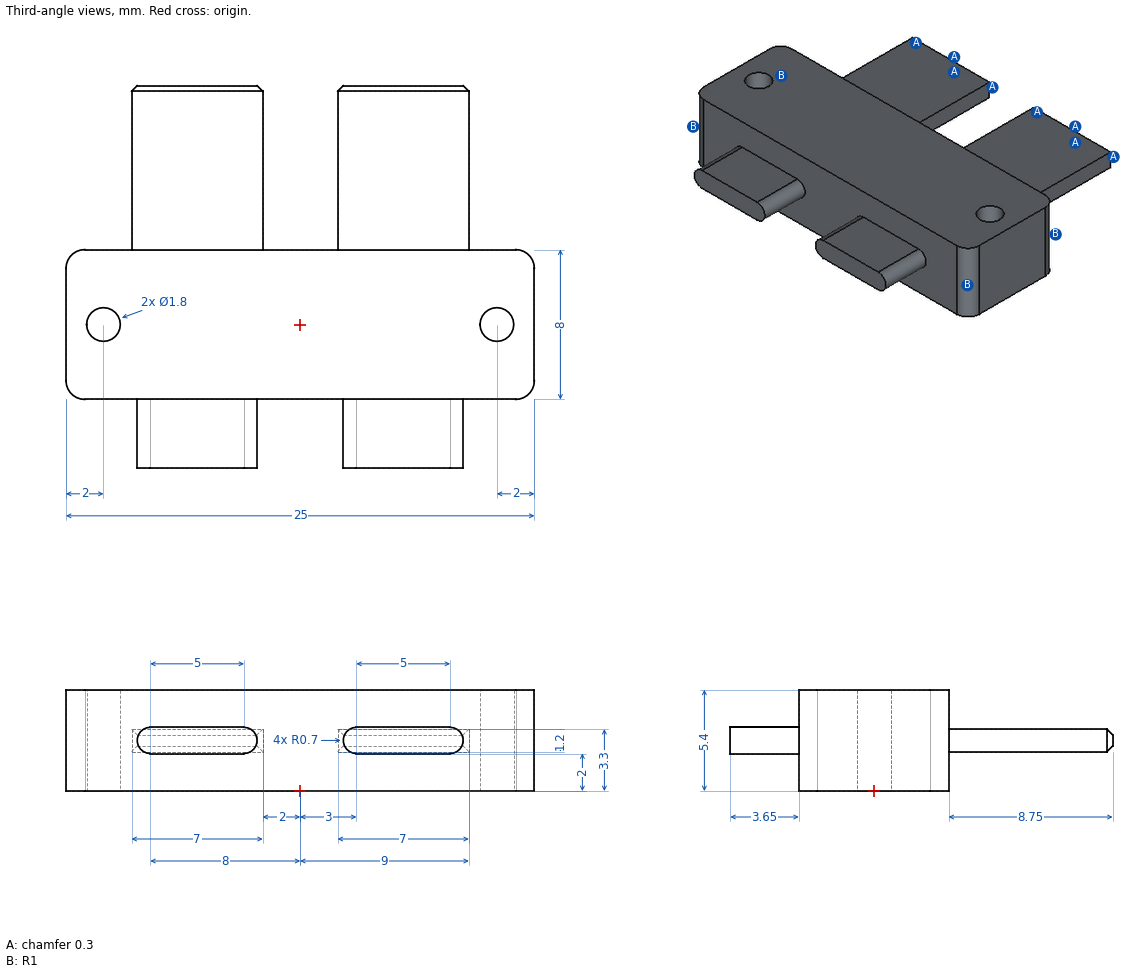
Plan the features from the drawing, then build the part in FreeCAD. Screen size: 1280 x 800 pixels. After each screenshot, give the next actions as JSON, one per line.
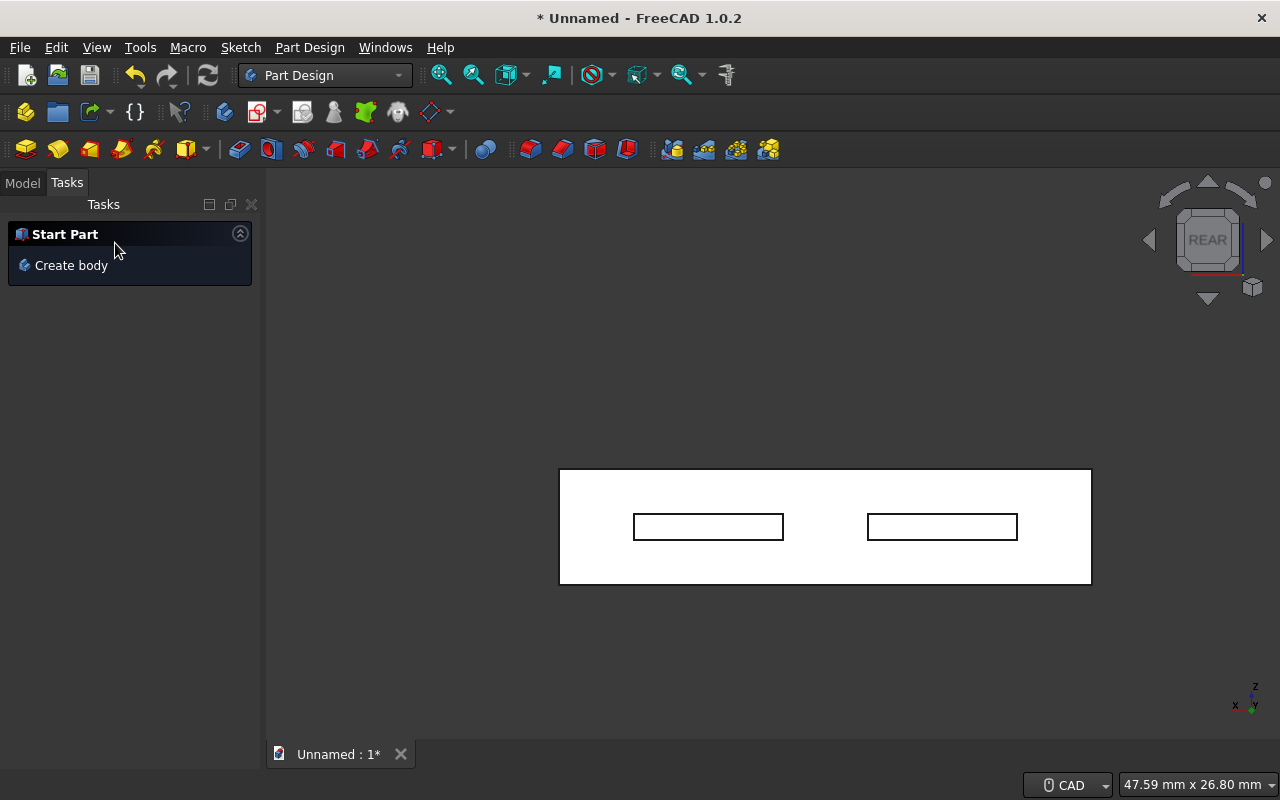
{"action": "left_click", "coordinate": [666, 526]}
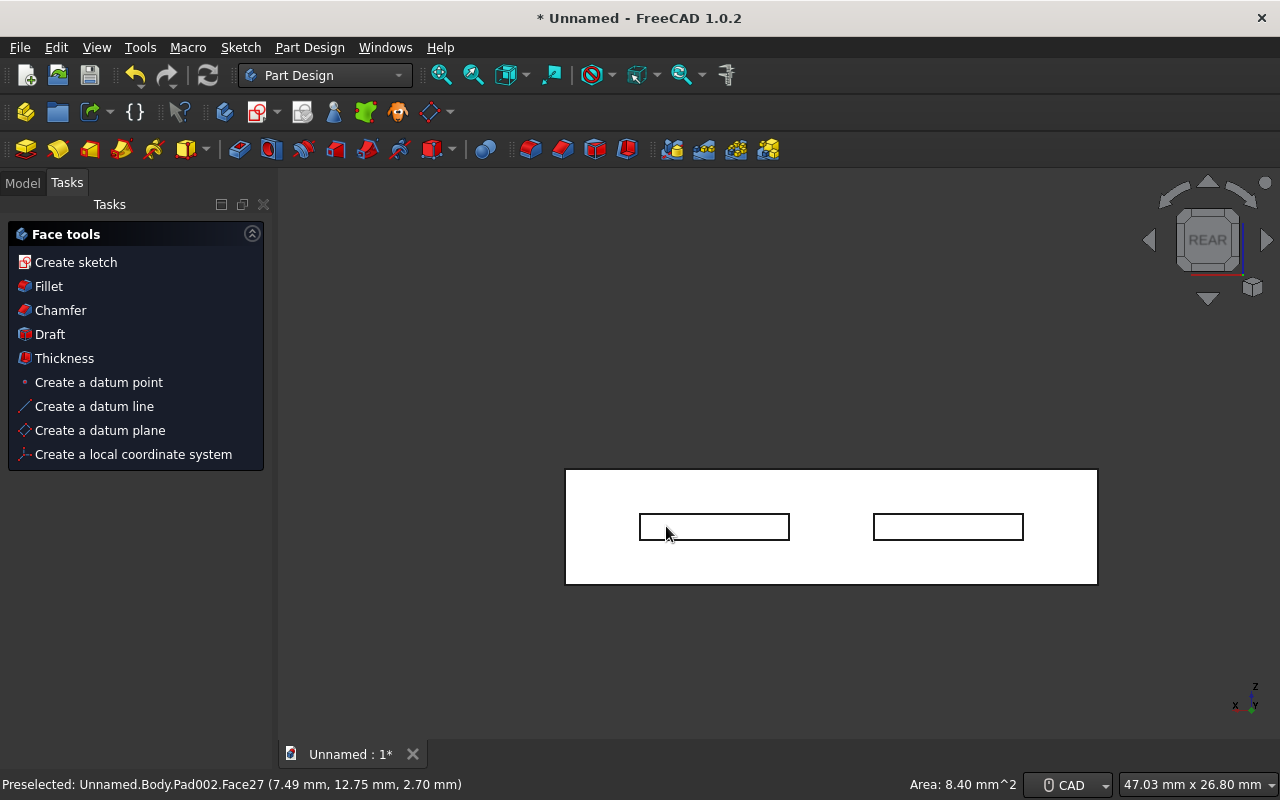
{"action": "left_click", "coordinate": [906, 526], "text": "ctrl"}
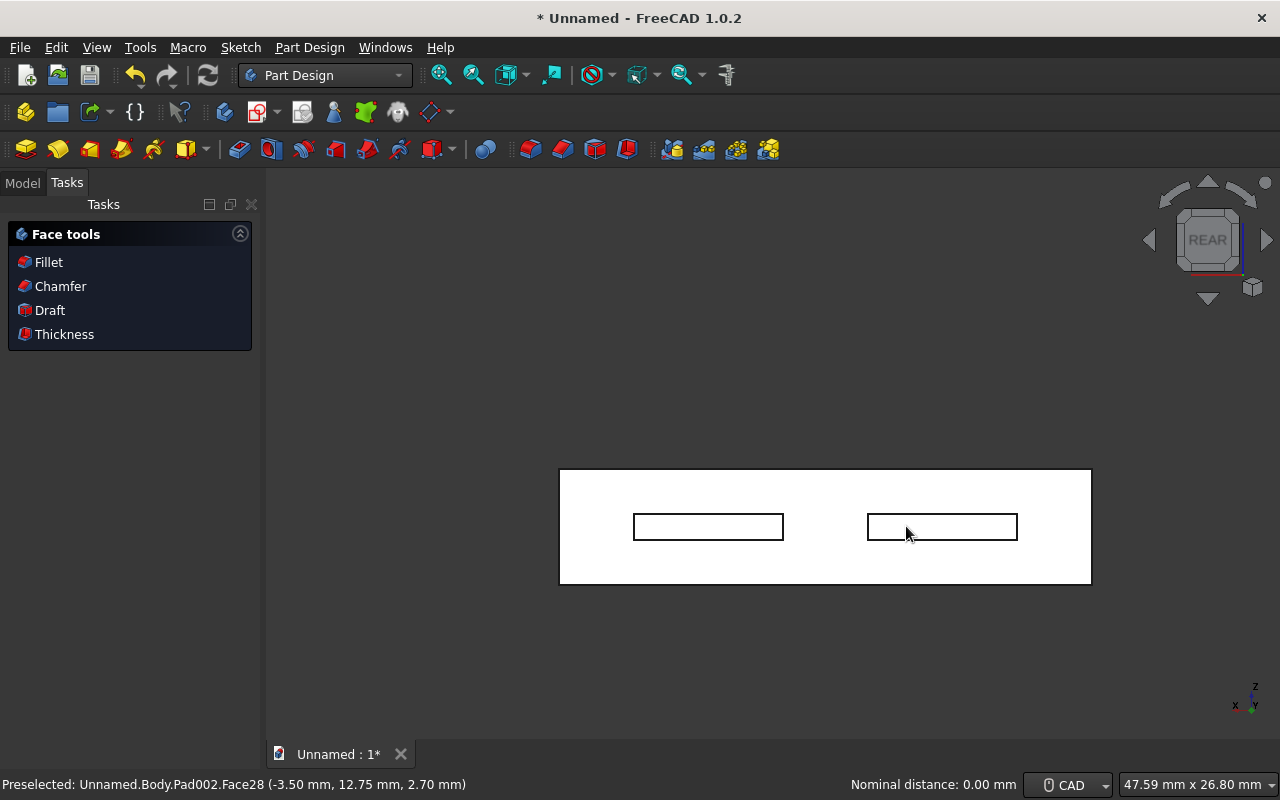
{"action": "left_click", "coordinate": [564, 150]}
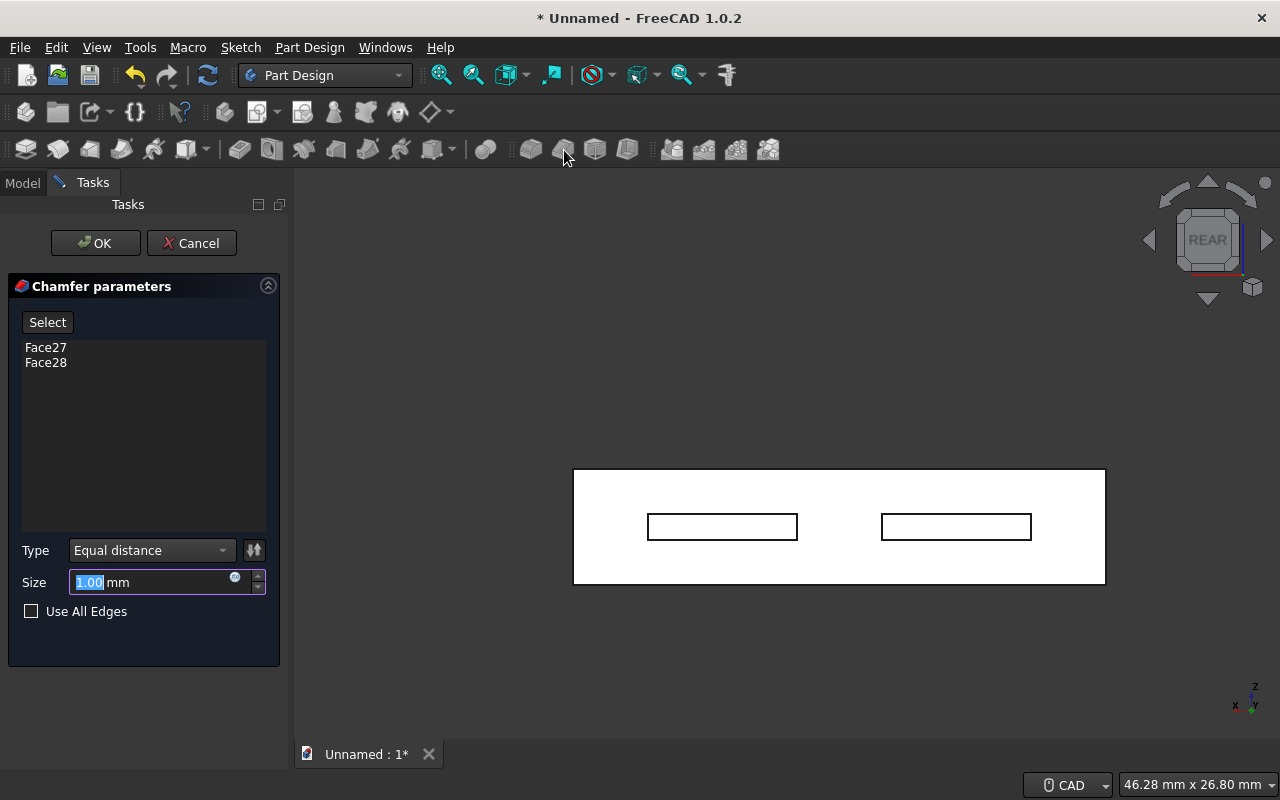
{"action": "type", "text": "0.3"}
{"action": "key", "text": "Tab"}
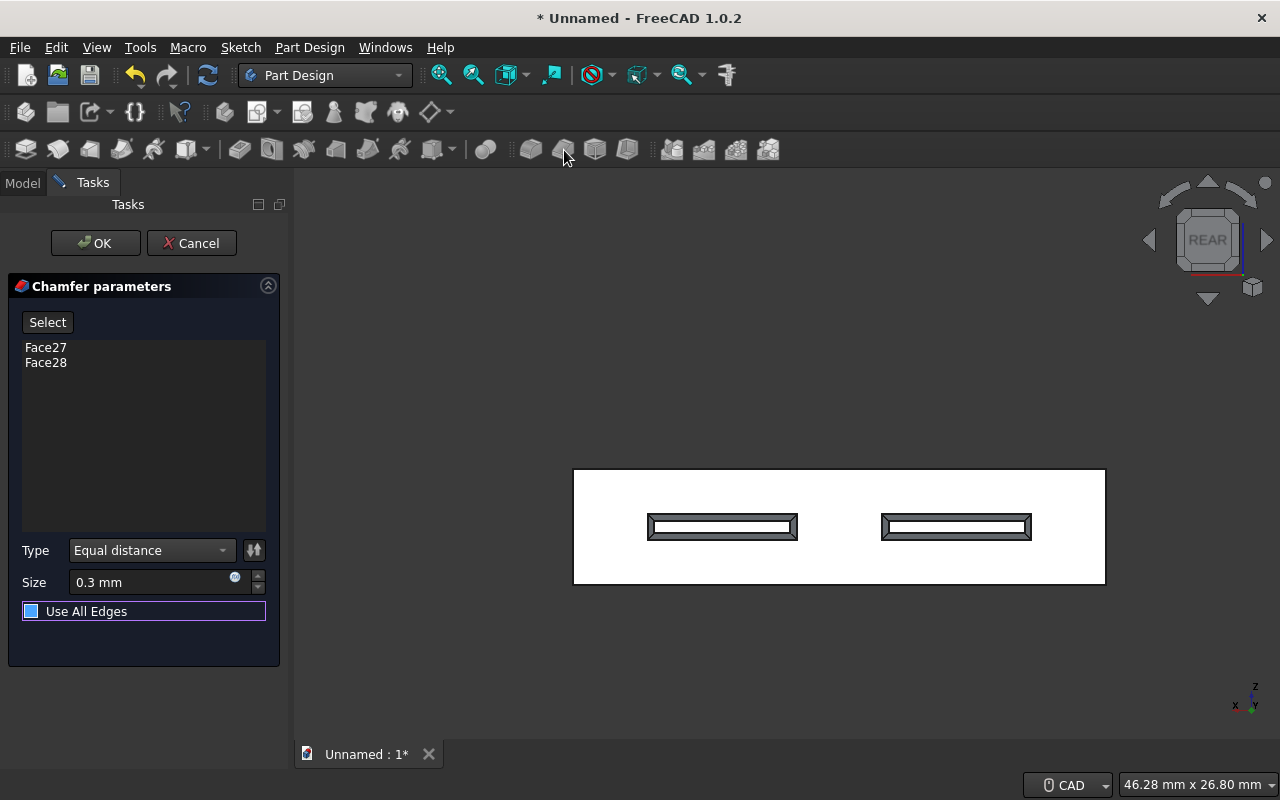
{"action": "left_click", "coordinate": [96, 243]}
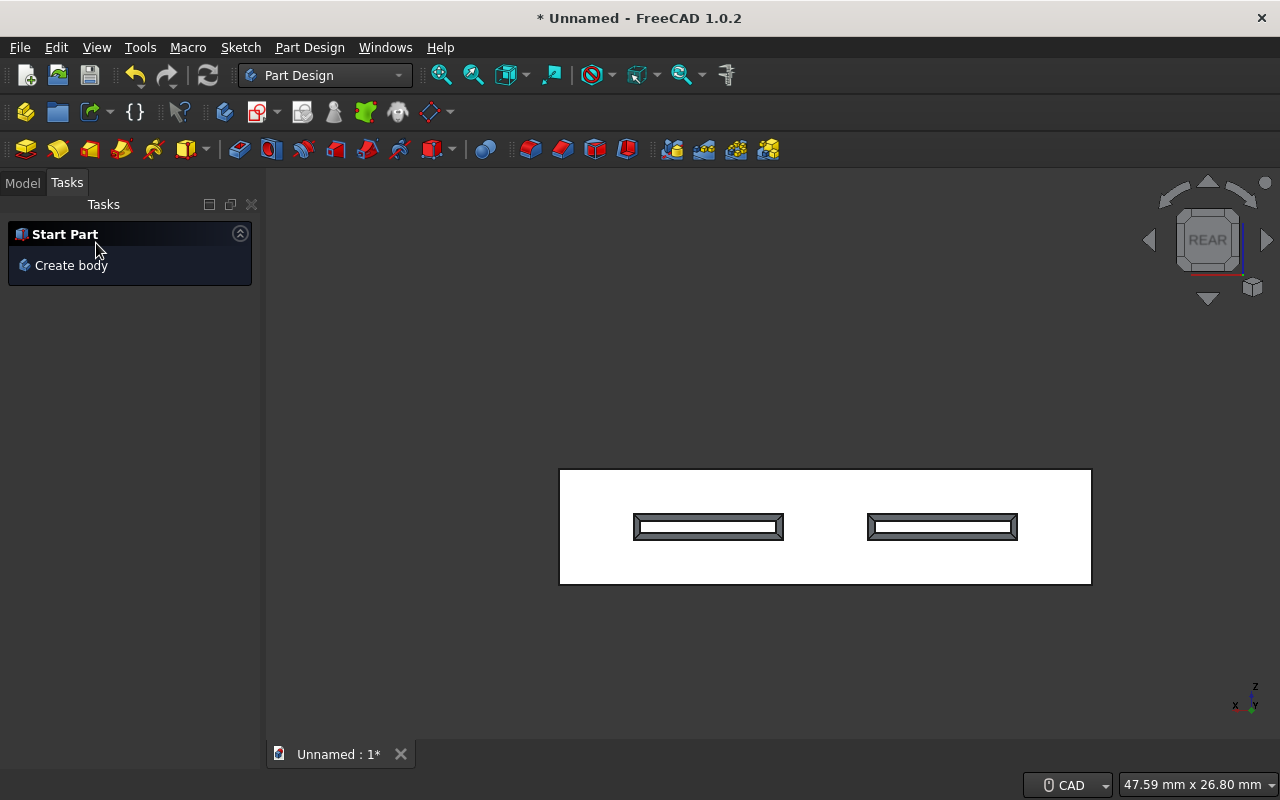
{"action": "left_click", "coordinate": [1092, 526]}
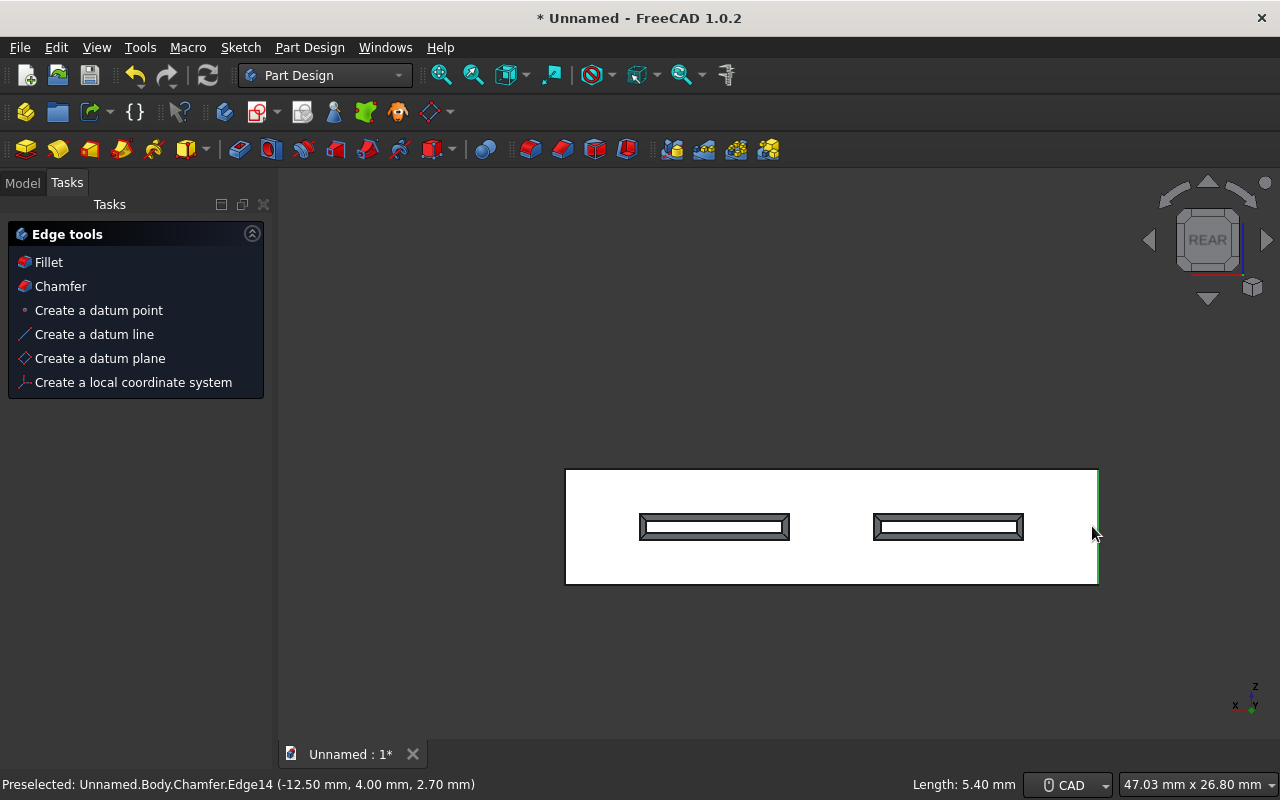
{"action": "key", "text": "0"}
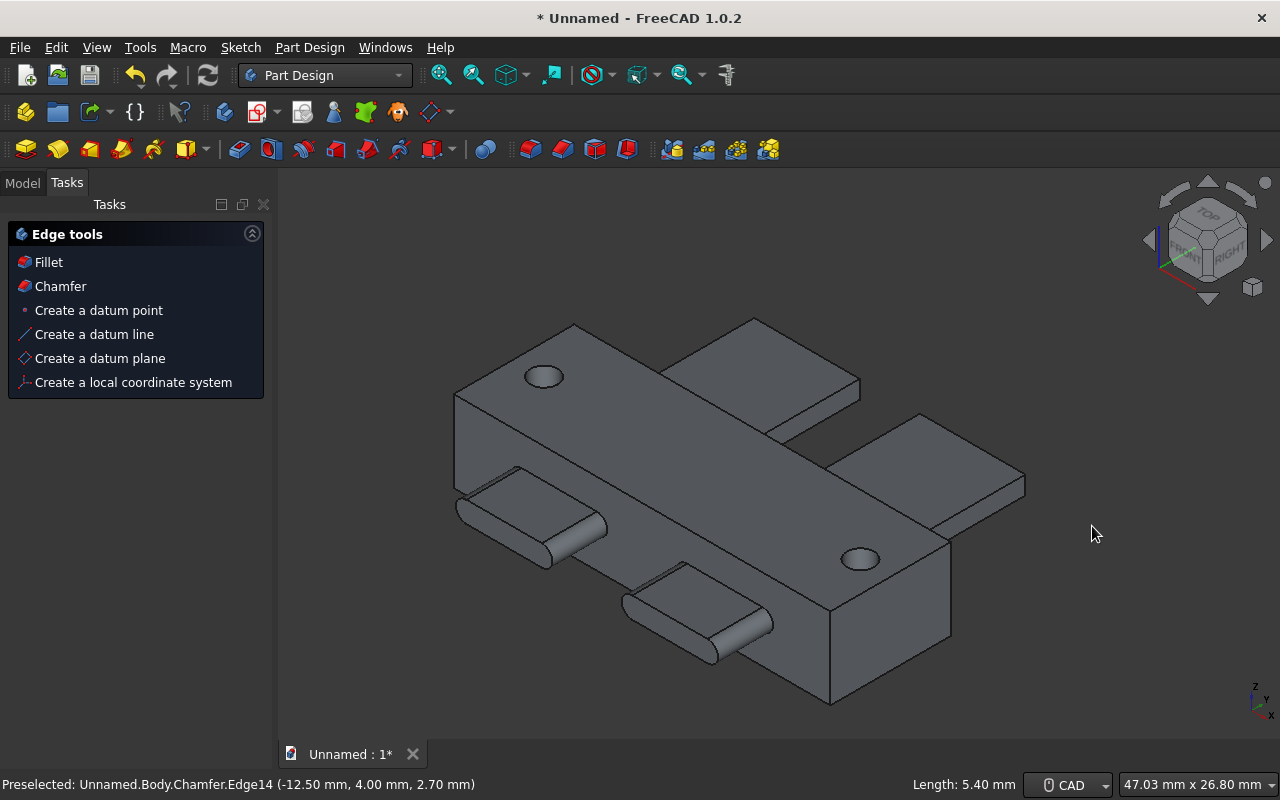
{"action": "left_click", "coordinate": [830, 657], "text": "ctrl"}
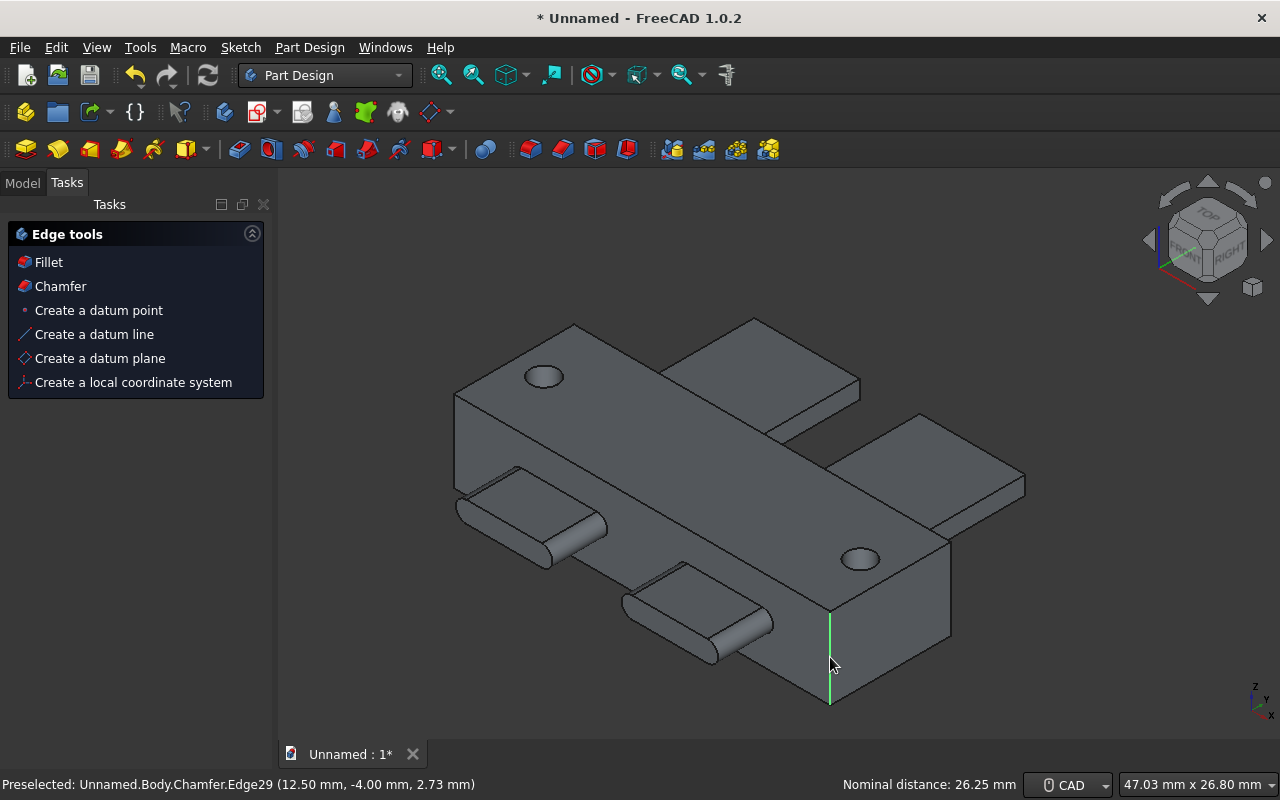
{"action": "key", "text": "2"}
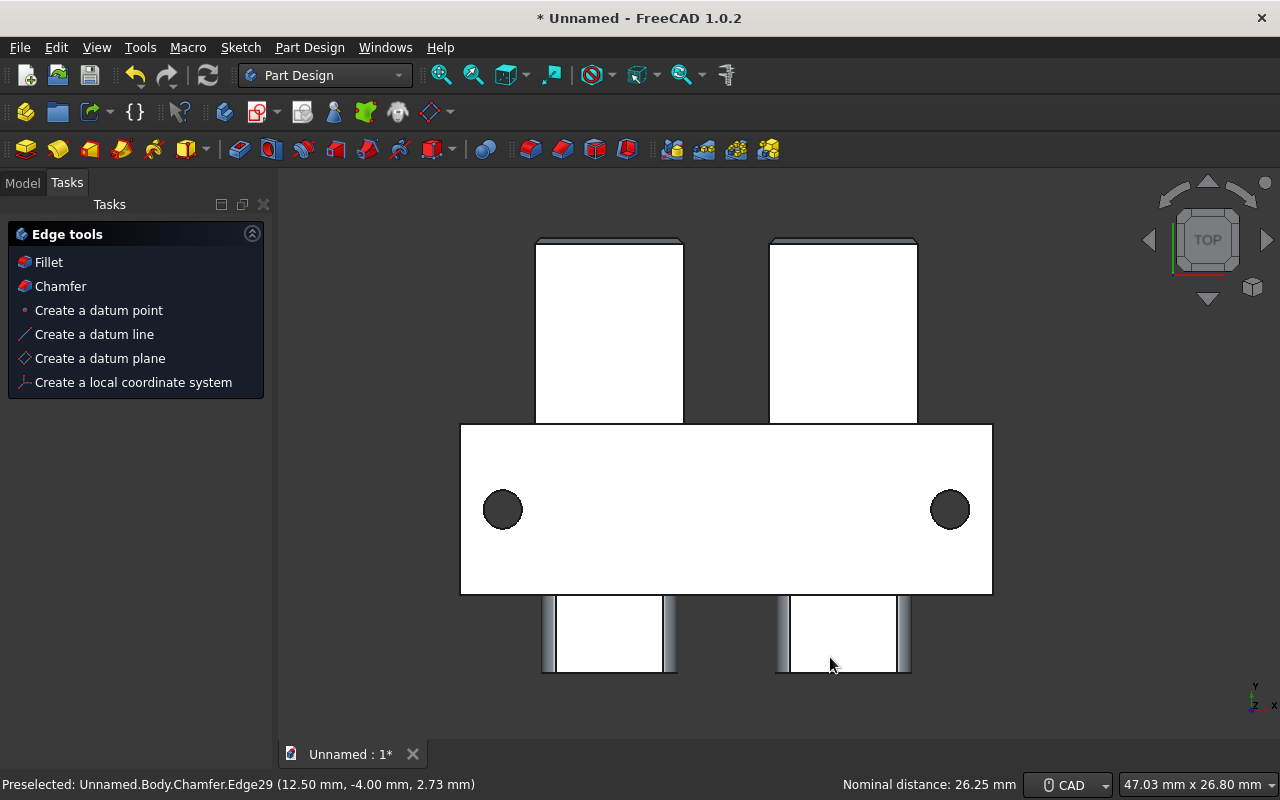
{"action": "key", "text": "1"}